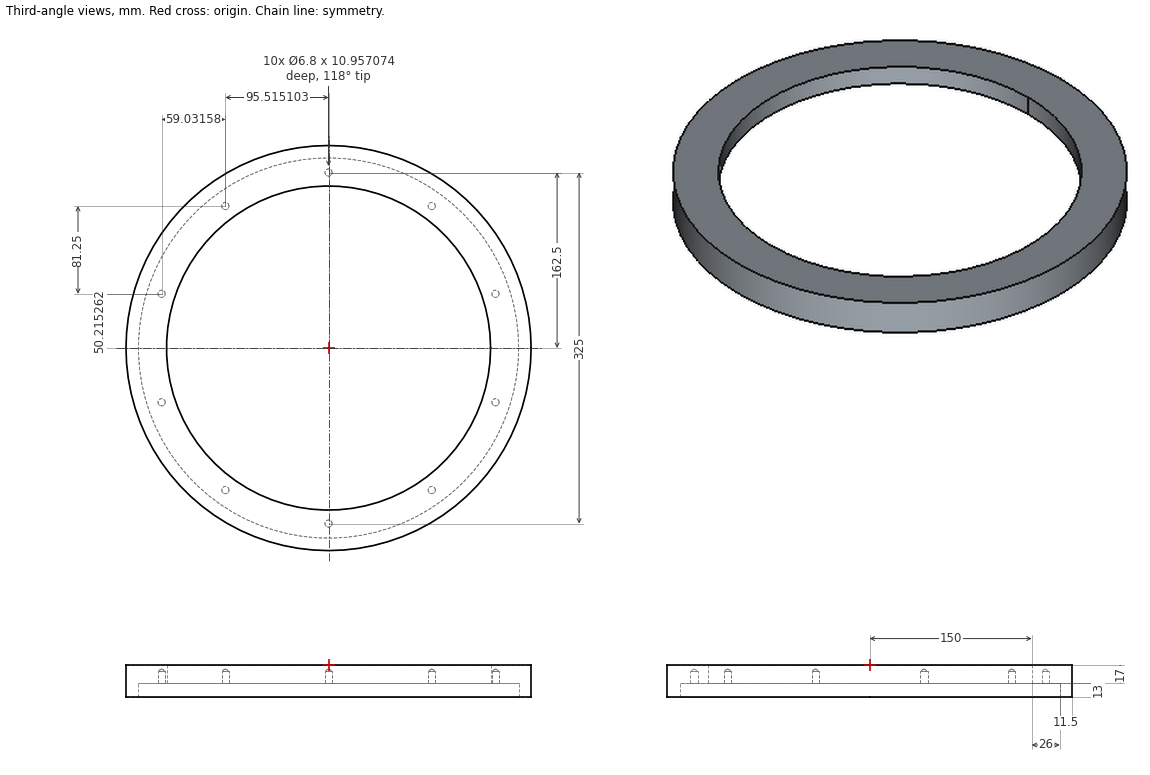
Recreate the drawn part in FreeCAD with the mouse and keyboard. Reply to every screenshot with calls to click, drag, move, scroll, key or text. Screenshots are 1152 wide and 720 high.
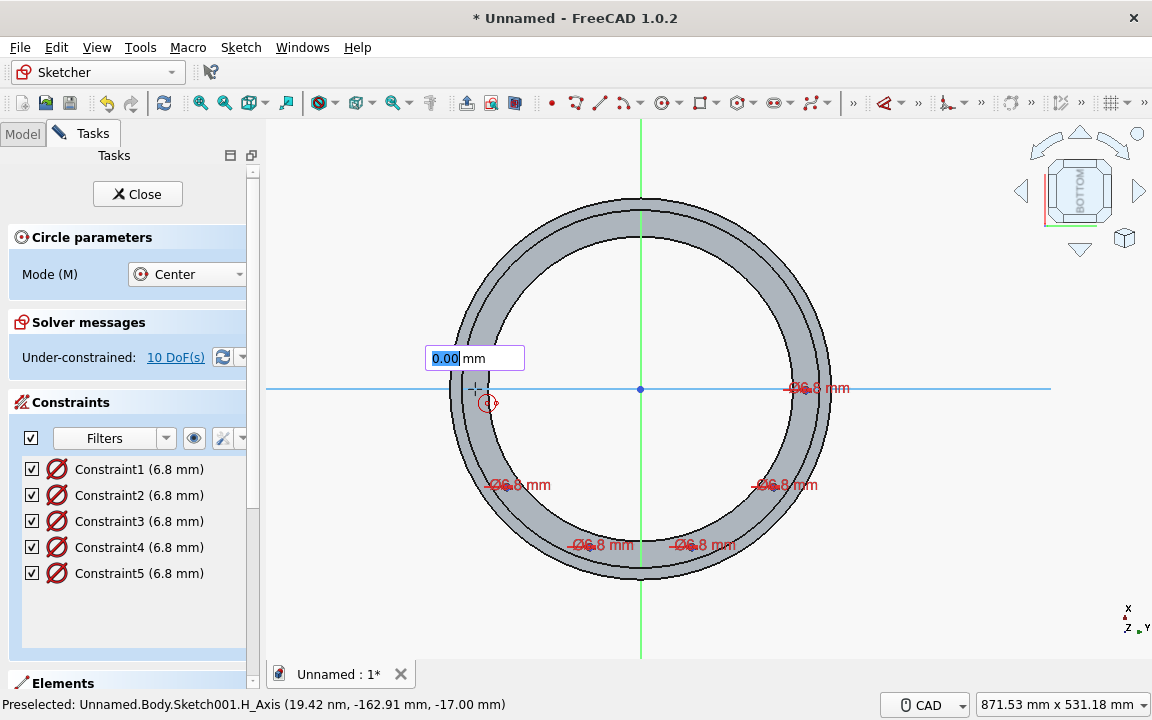
scroll(474, 392, up, 8)
move(474, 392)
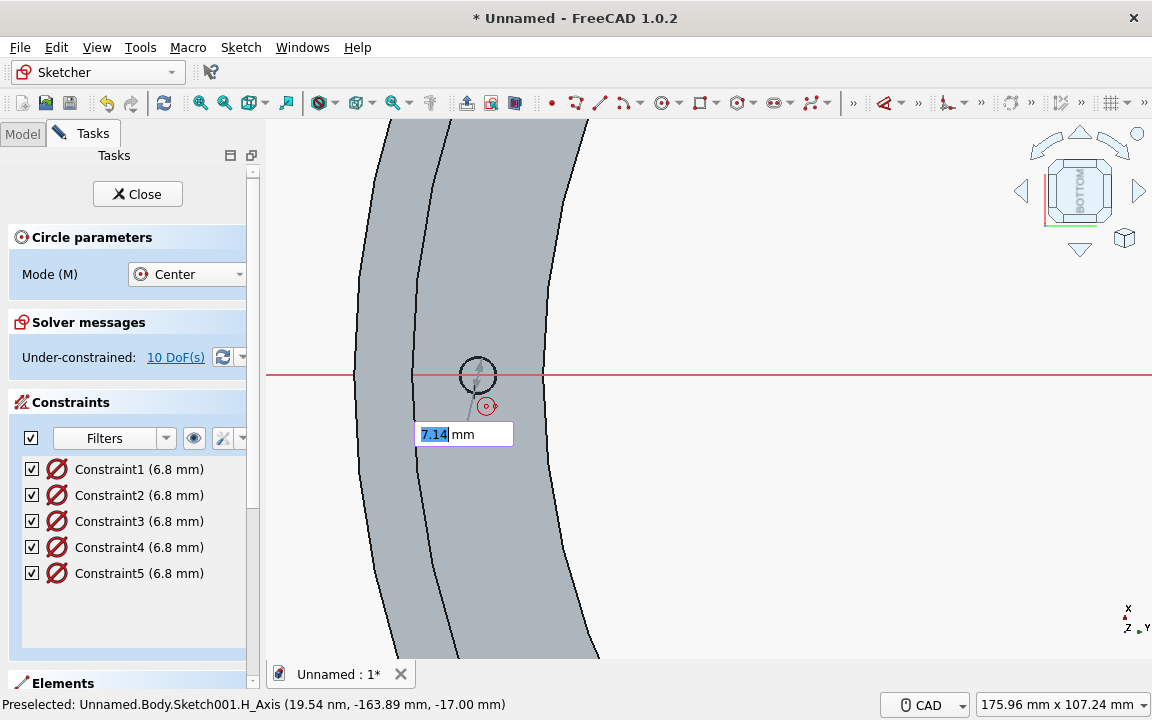
text(6.8)
key(Return)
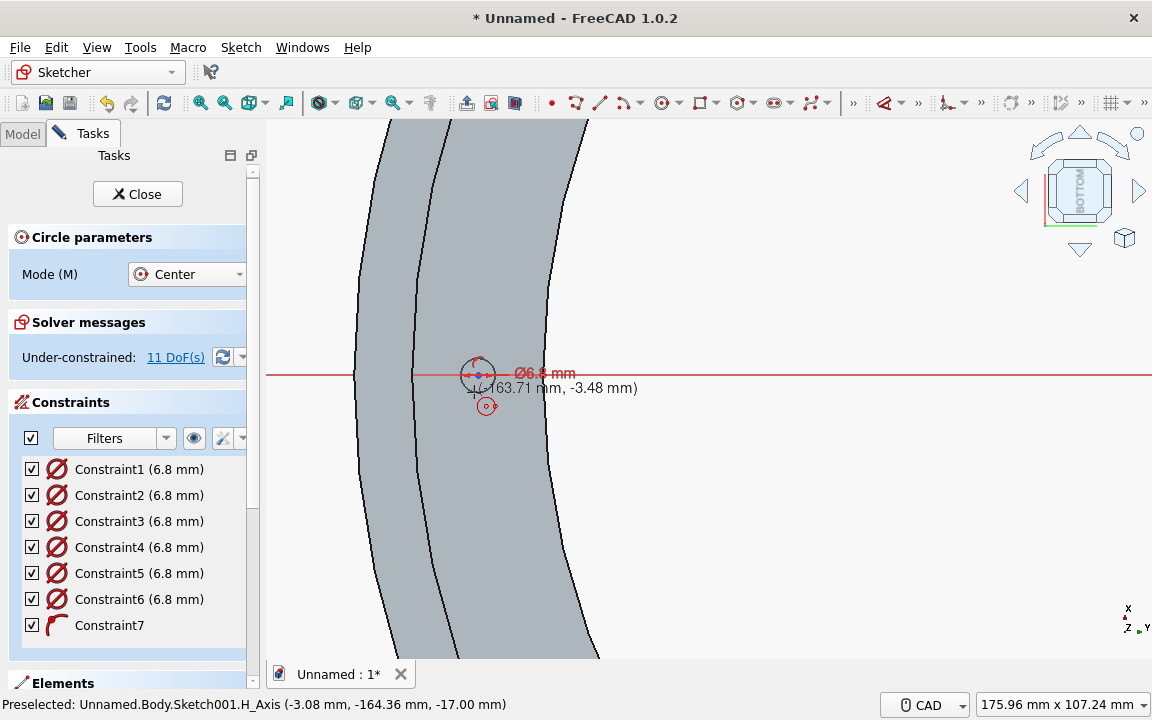
scroll(474, 392, down, 8)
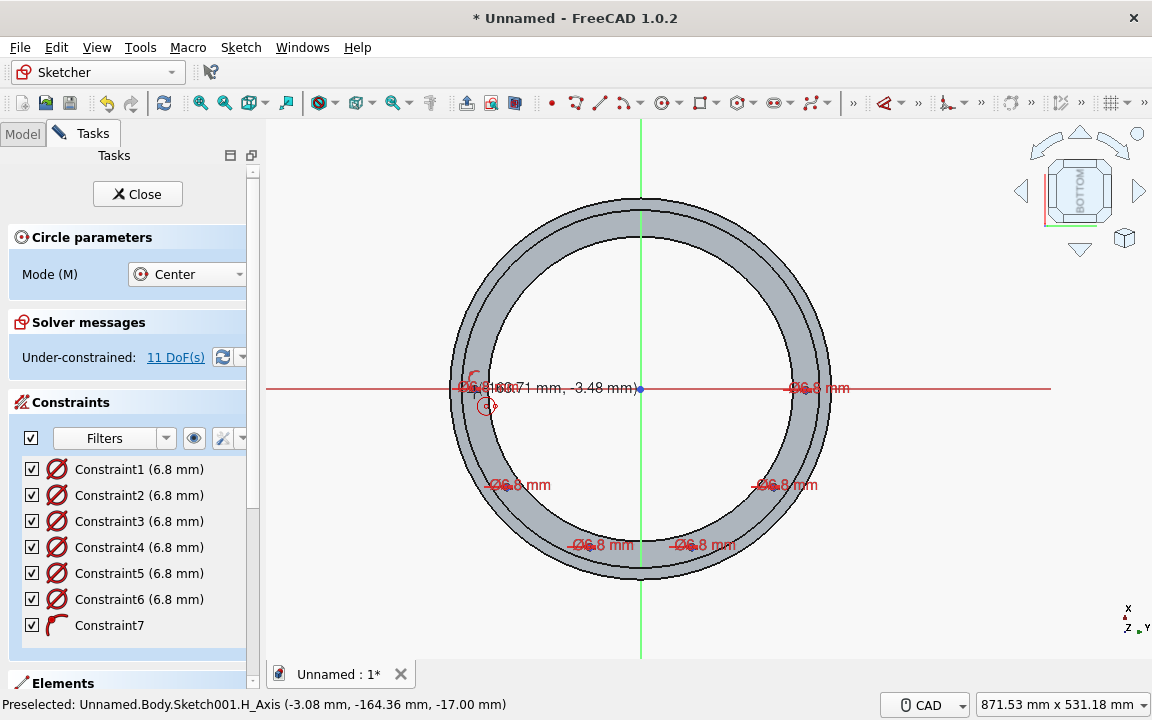
scroll(507, 292, up, 10)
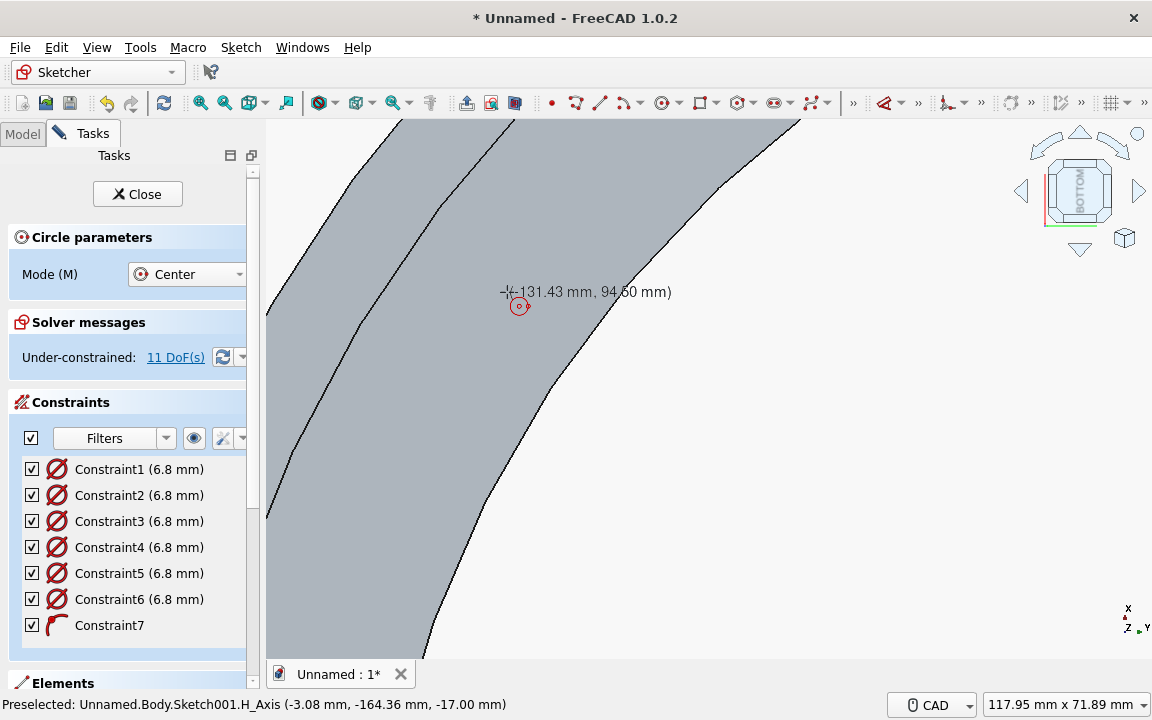
scroll(507, 292, down, 10)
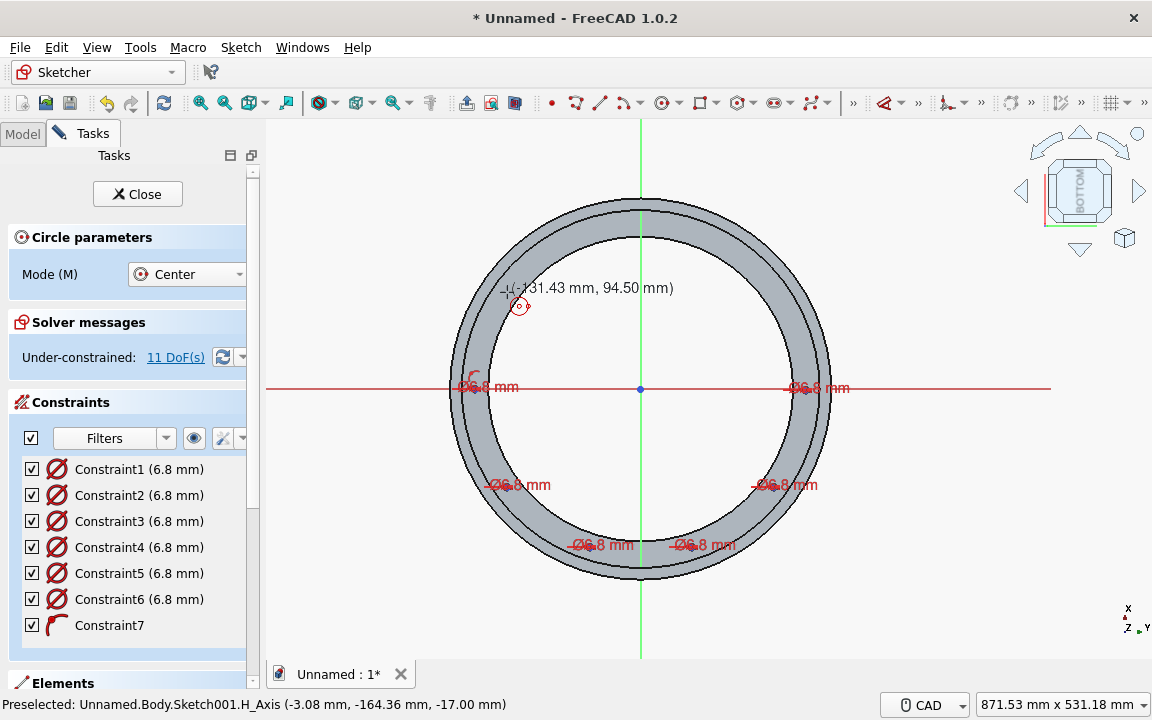
click(507, 292)
move(509, 290)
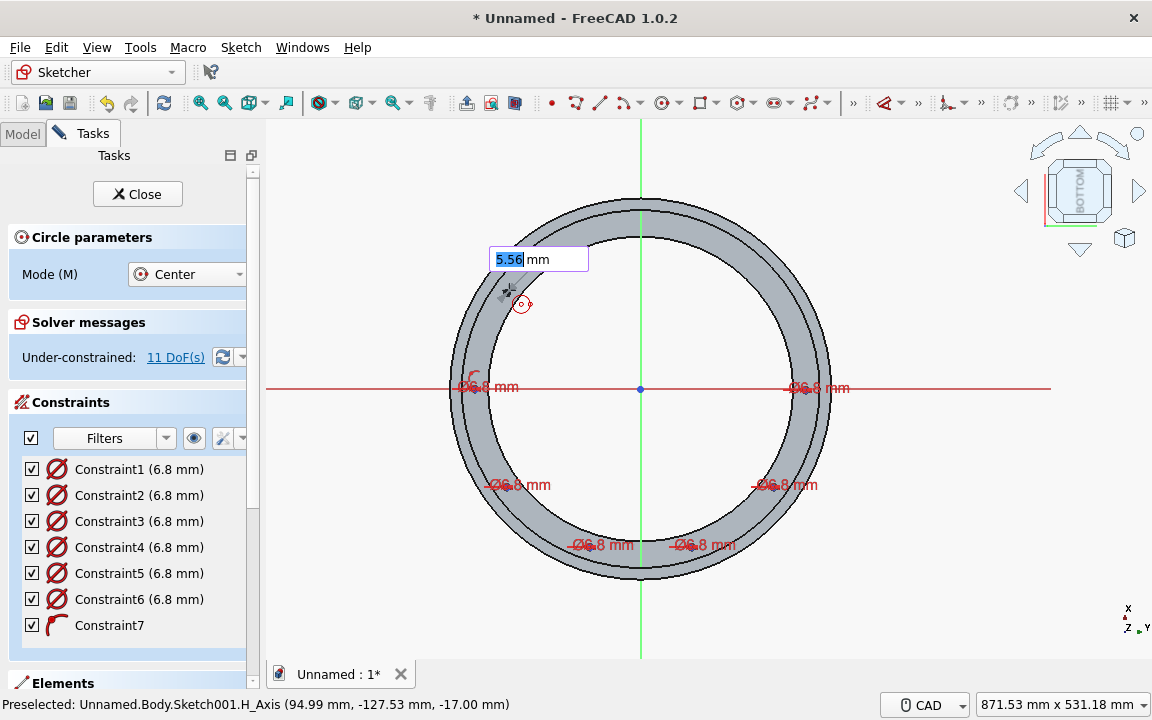
text(6.8)
key(Return)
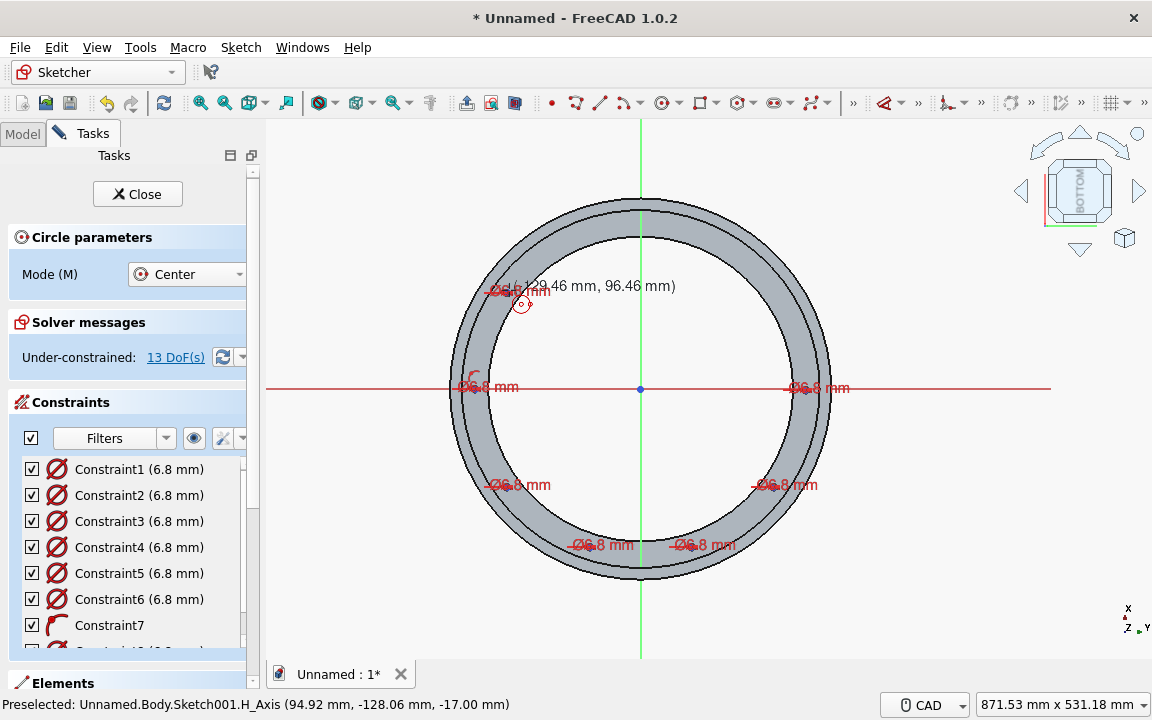
scroll(590, 232, up, 10)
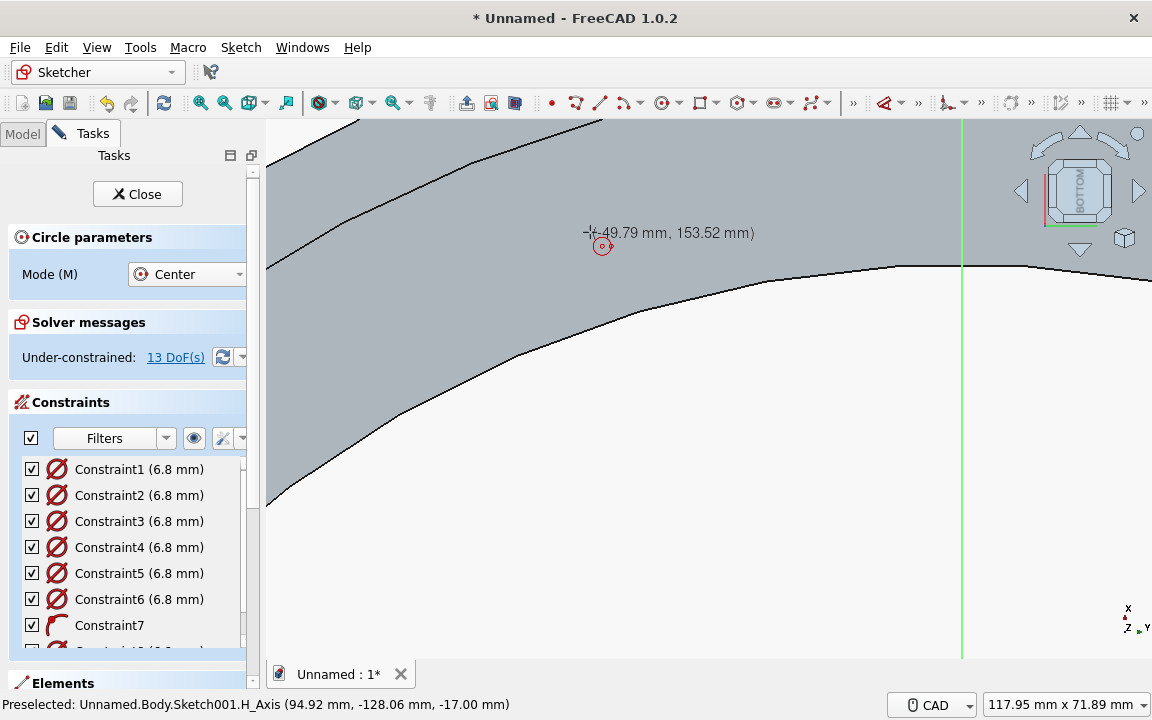
scroll(590, 232, down, 10)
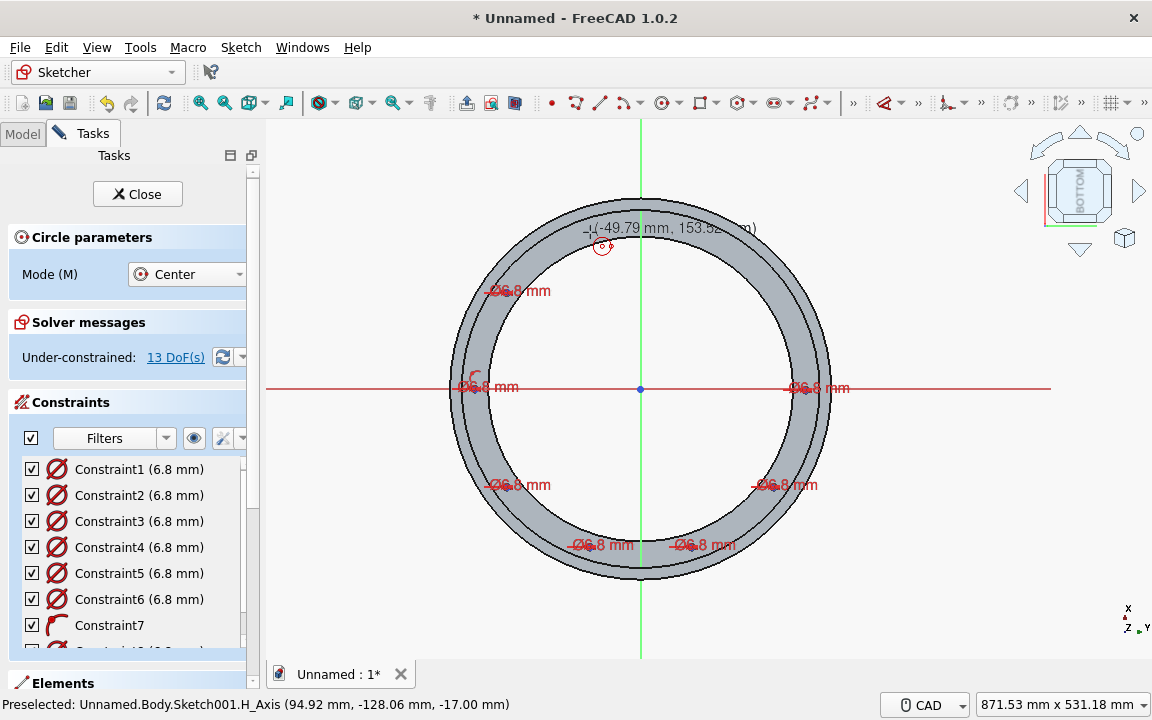
click(590, 232)
move(592, 230)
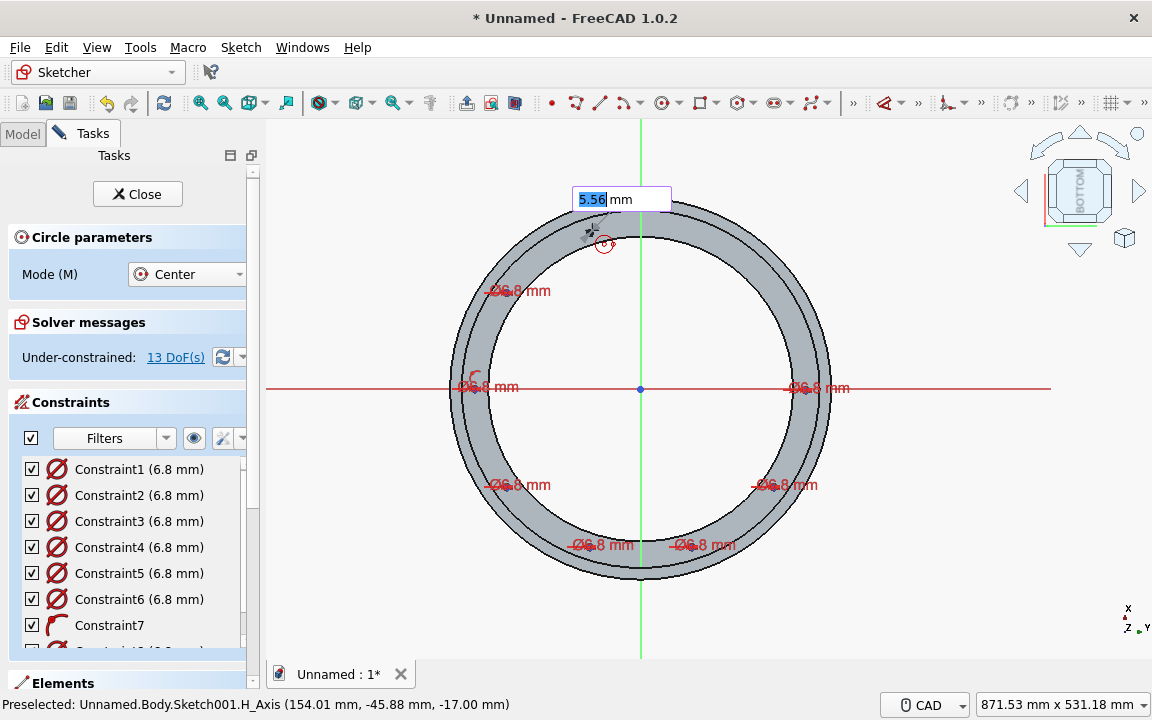
text(6.8)
key(Return)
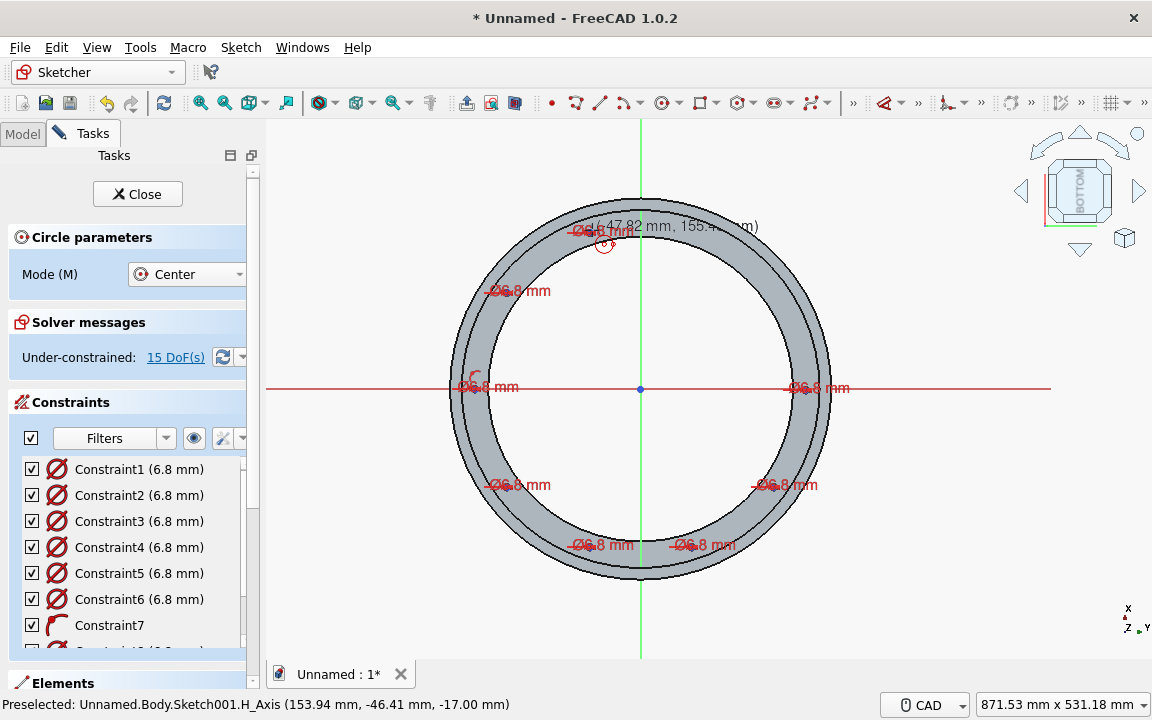
scroll(692, 232, up, 10)